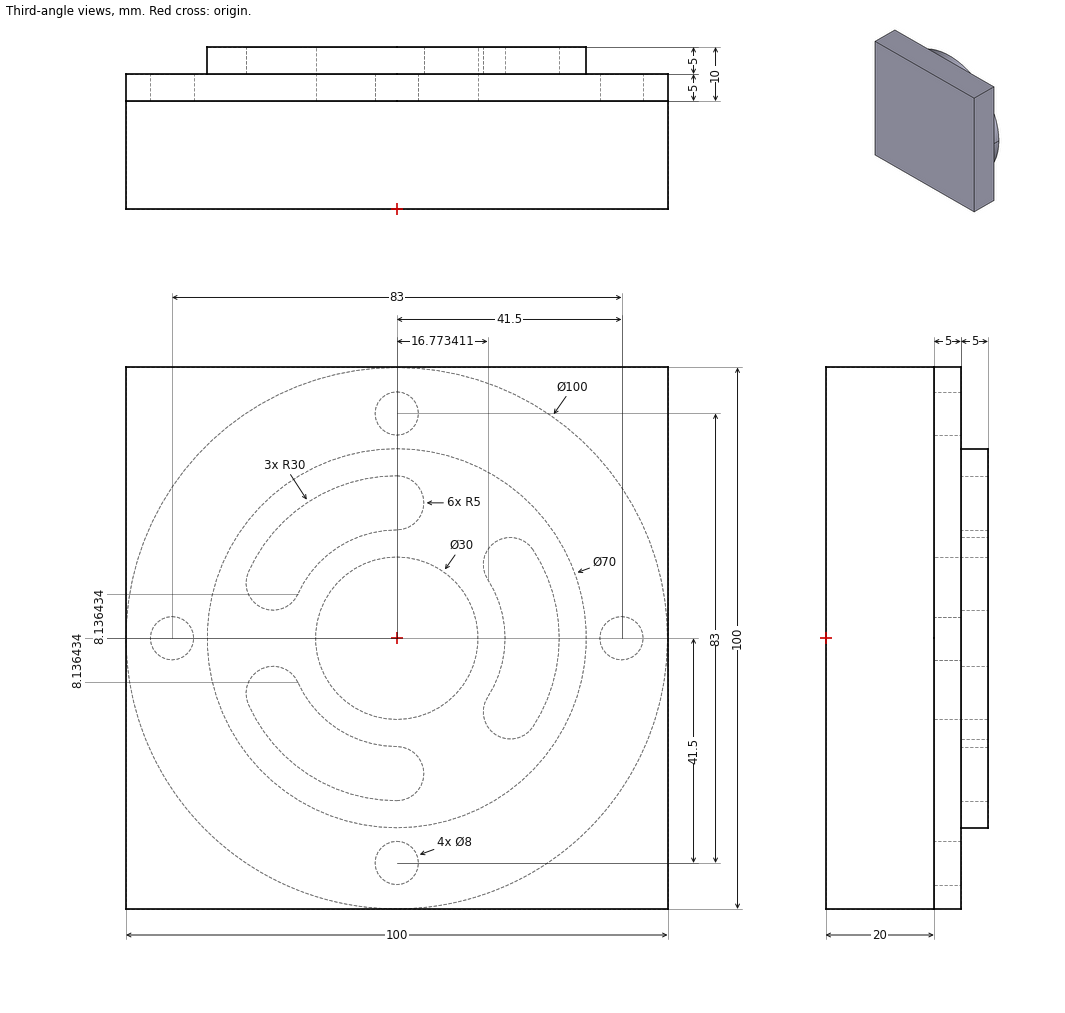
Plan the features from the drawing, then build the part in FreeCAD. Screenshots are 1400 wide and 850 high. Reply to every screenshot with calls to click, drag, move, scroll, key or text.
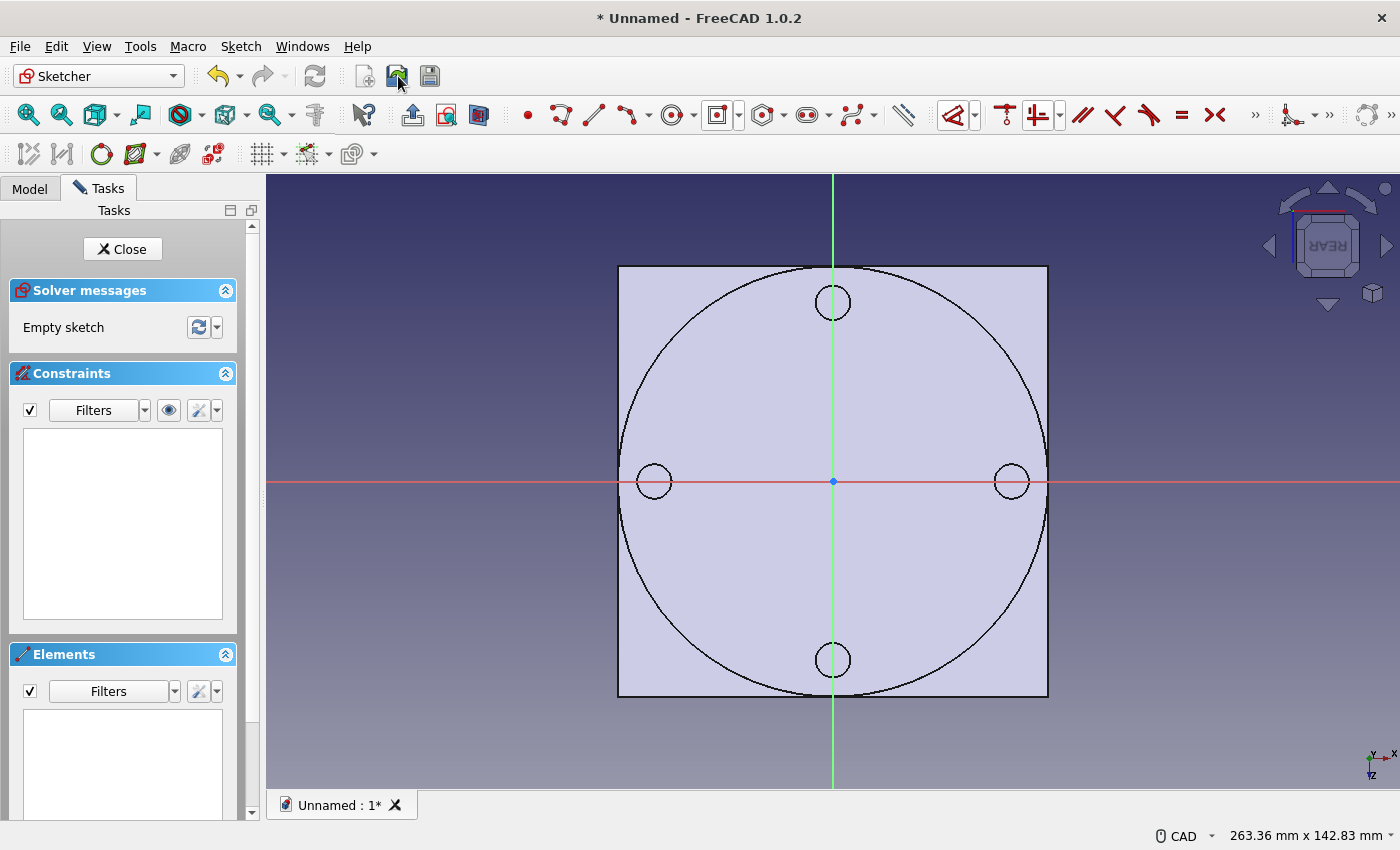
click(672, 116)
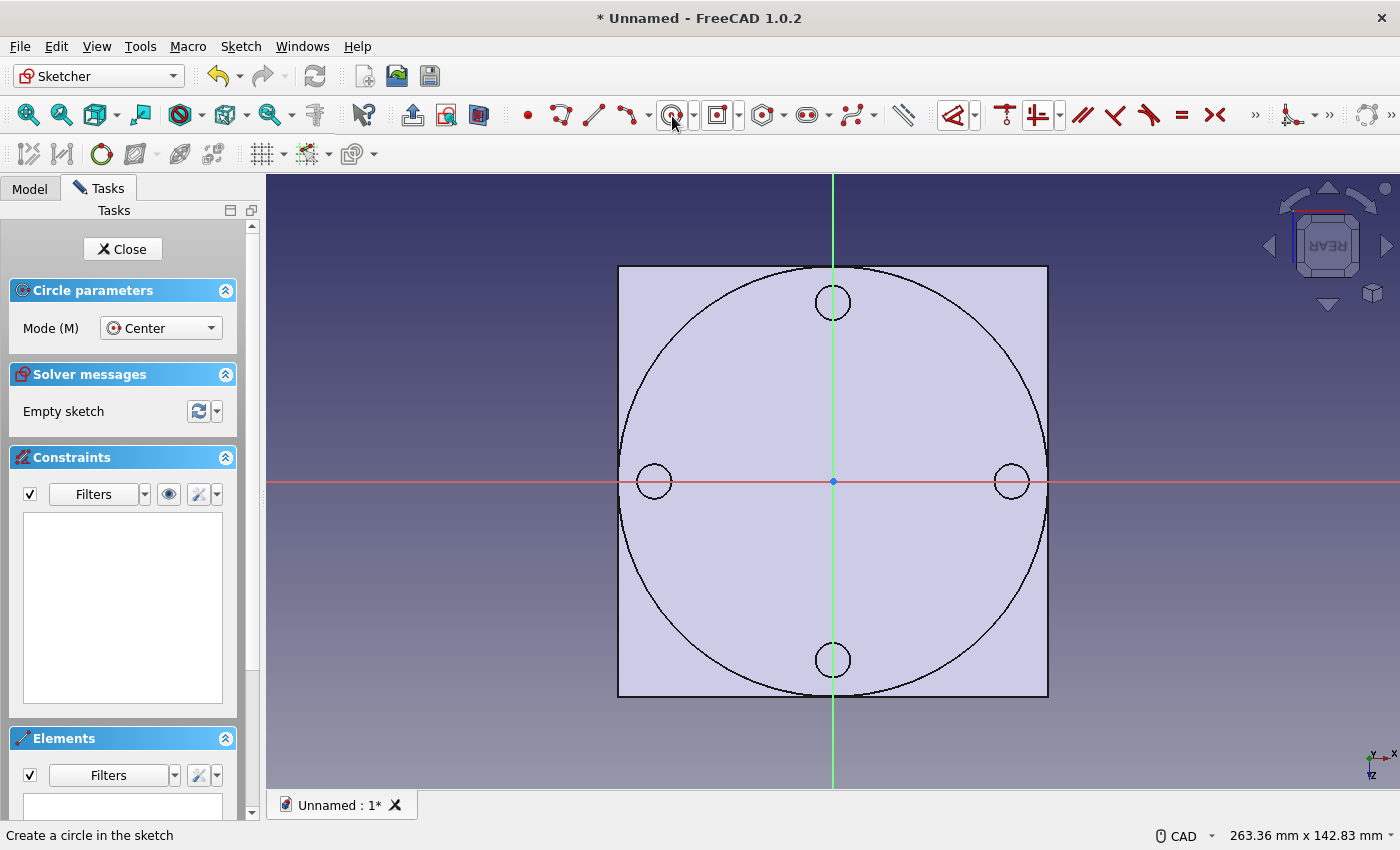
click(833, 481)
move(940, 375)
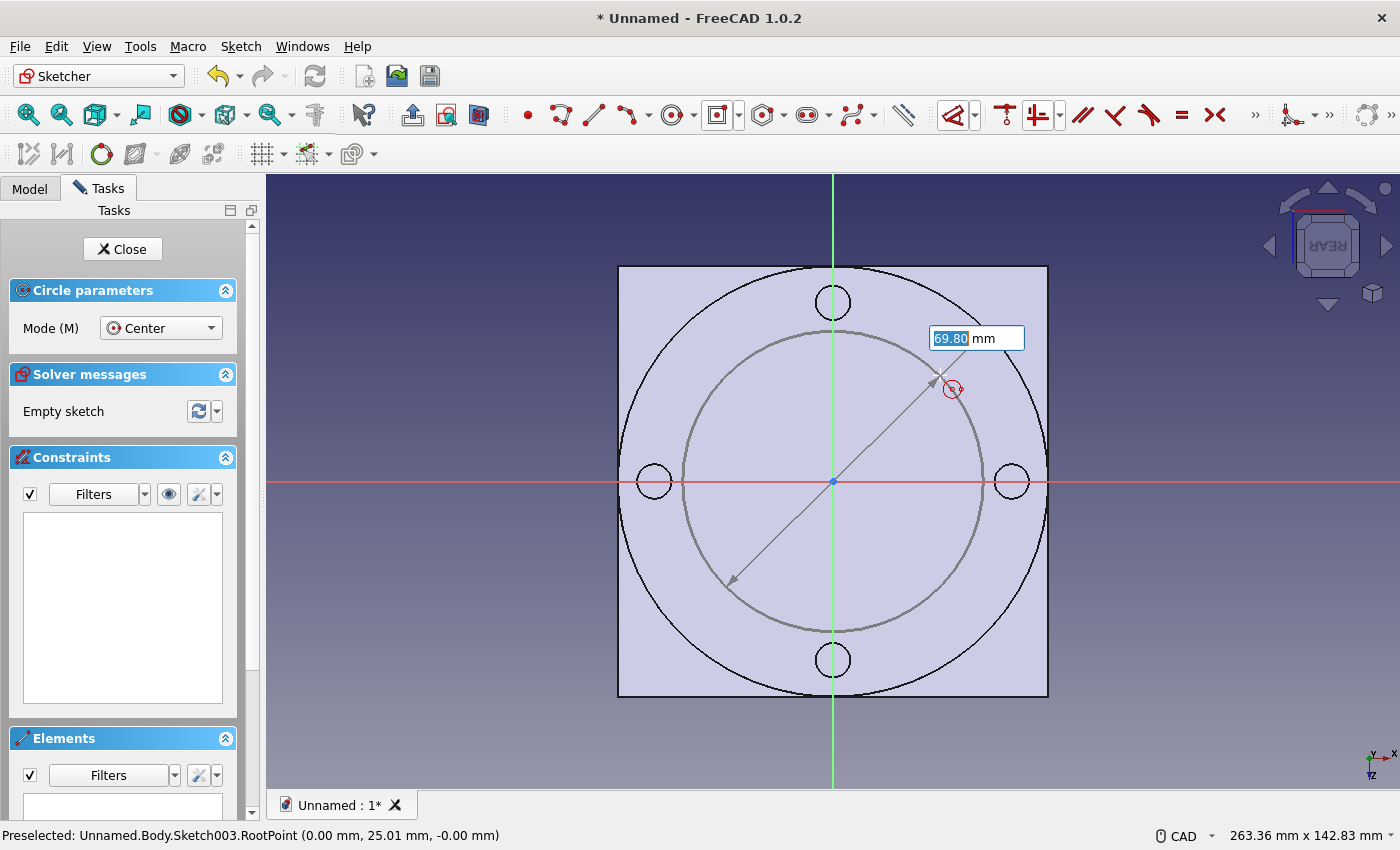
text(70)
key(Return)
key(Escape)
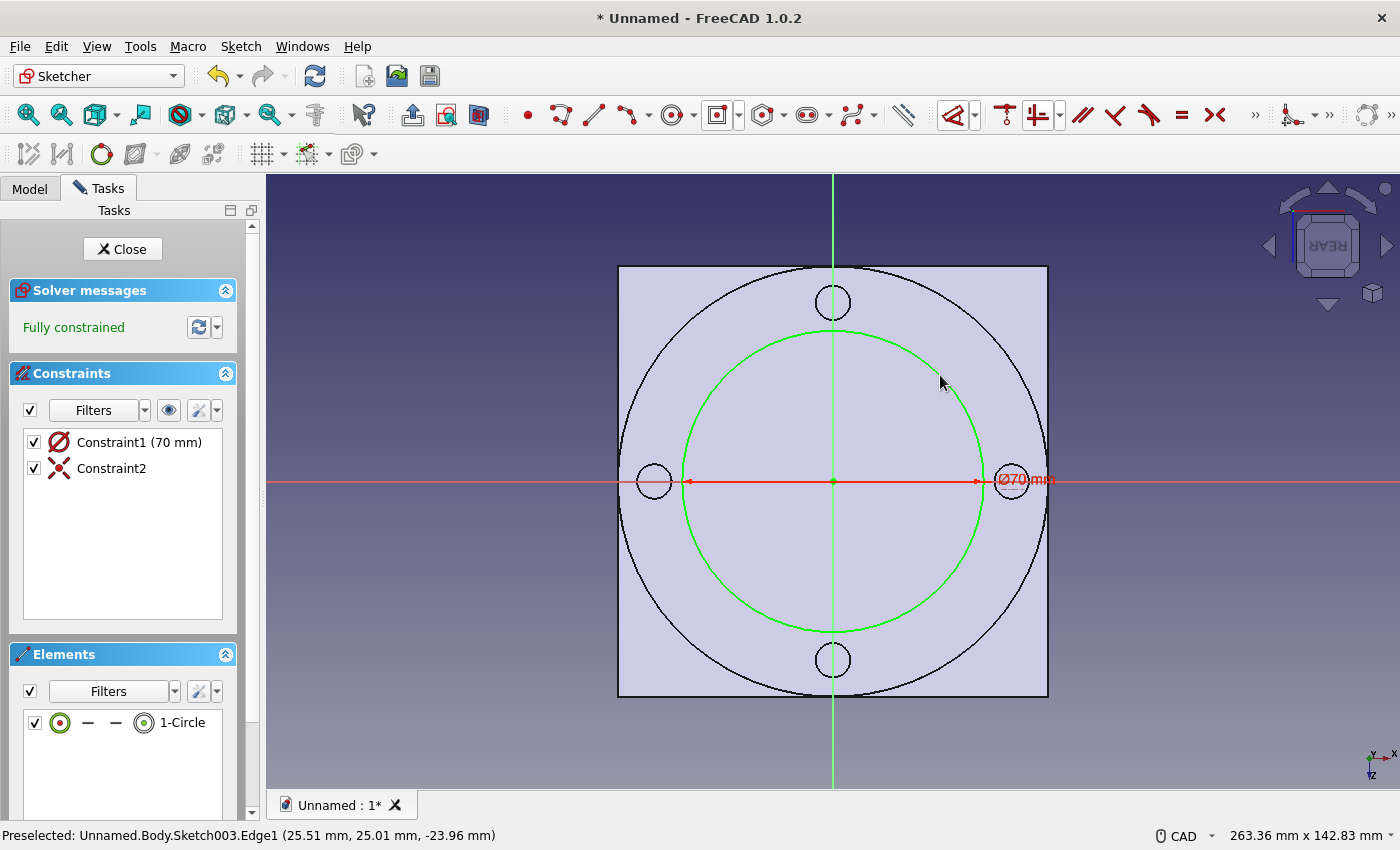
click(123, 249)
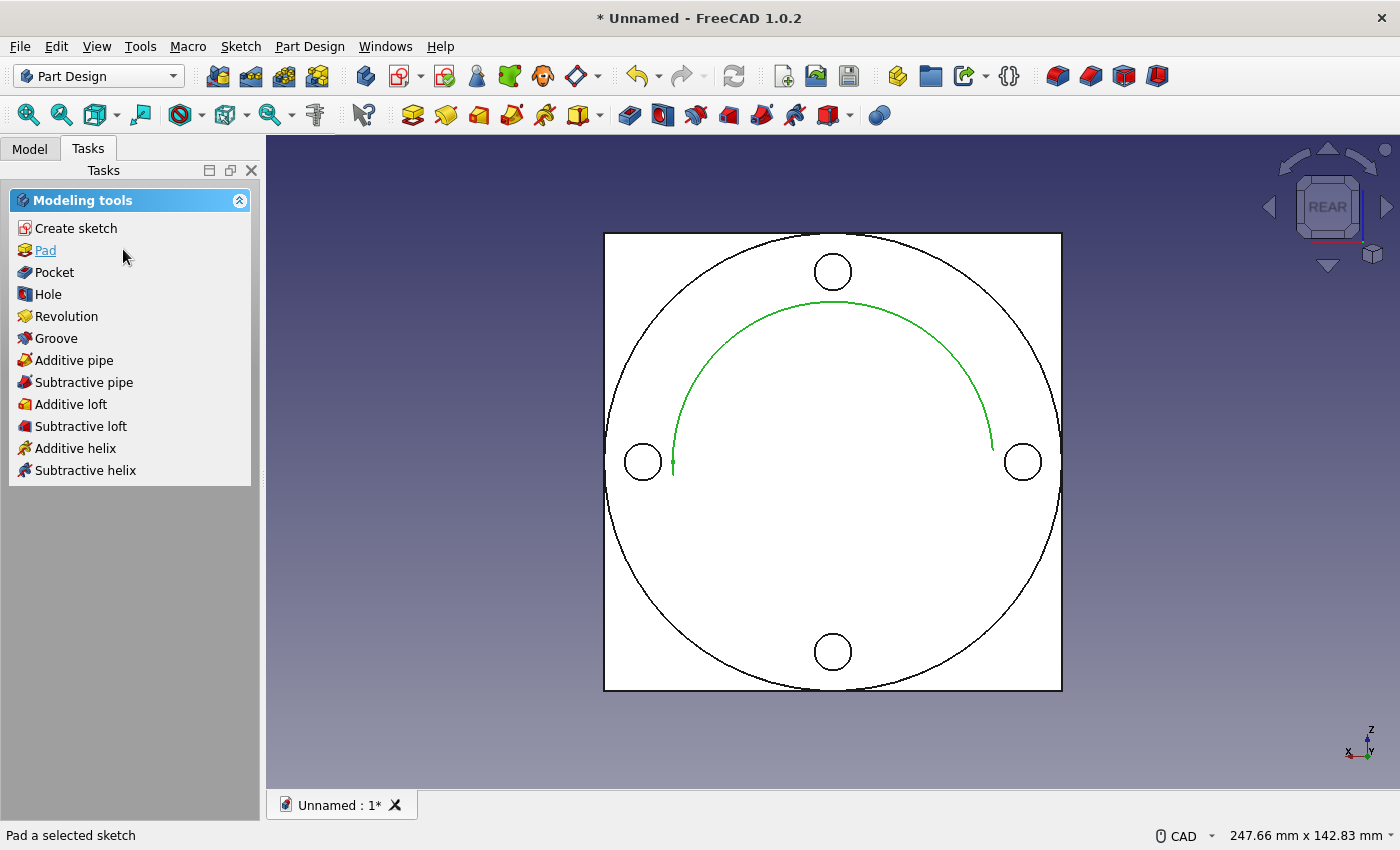
click(413, 116)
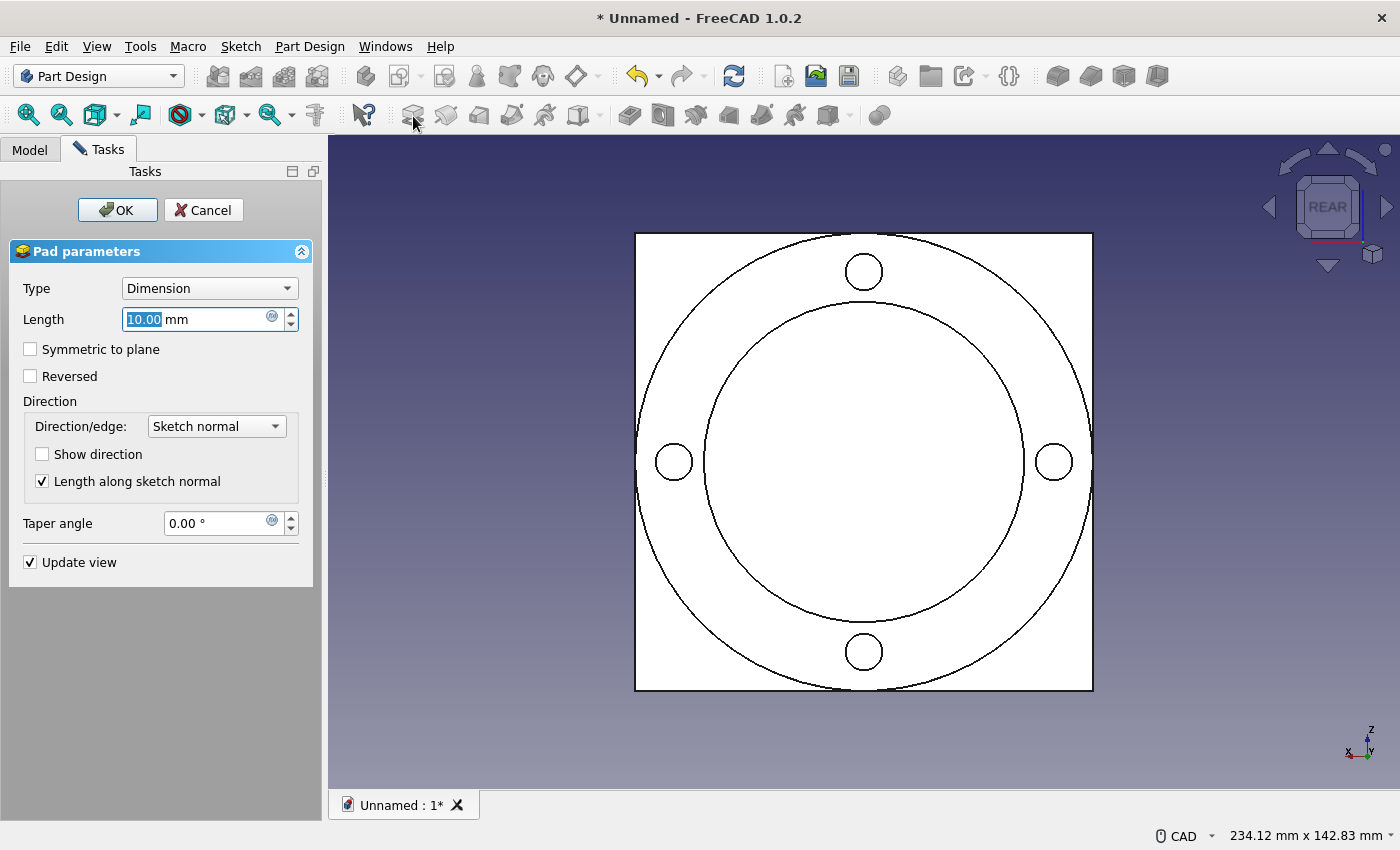
text(5)
key(Tab)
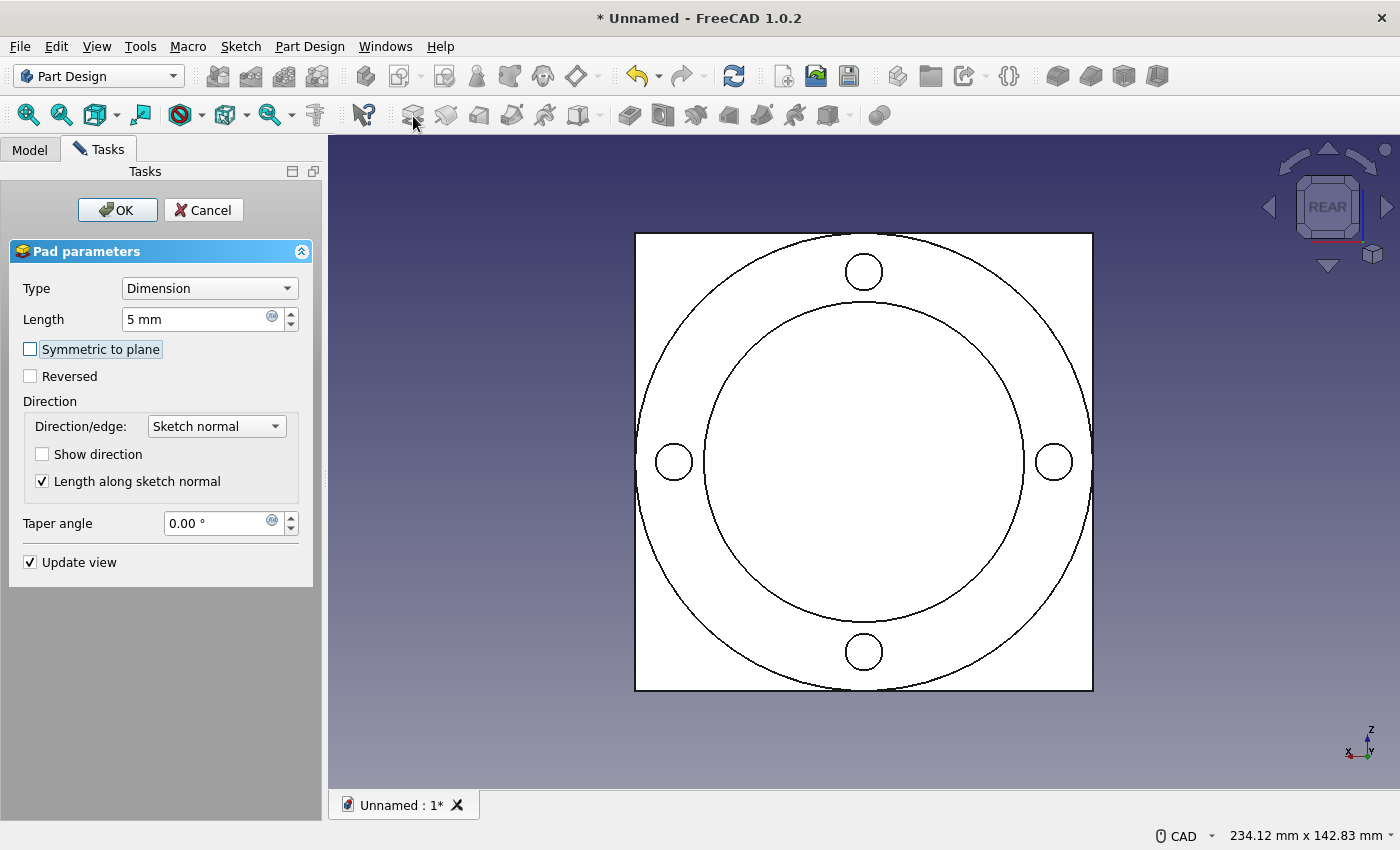
click(118, 210)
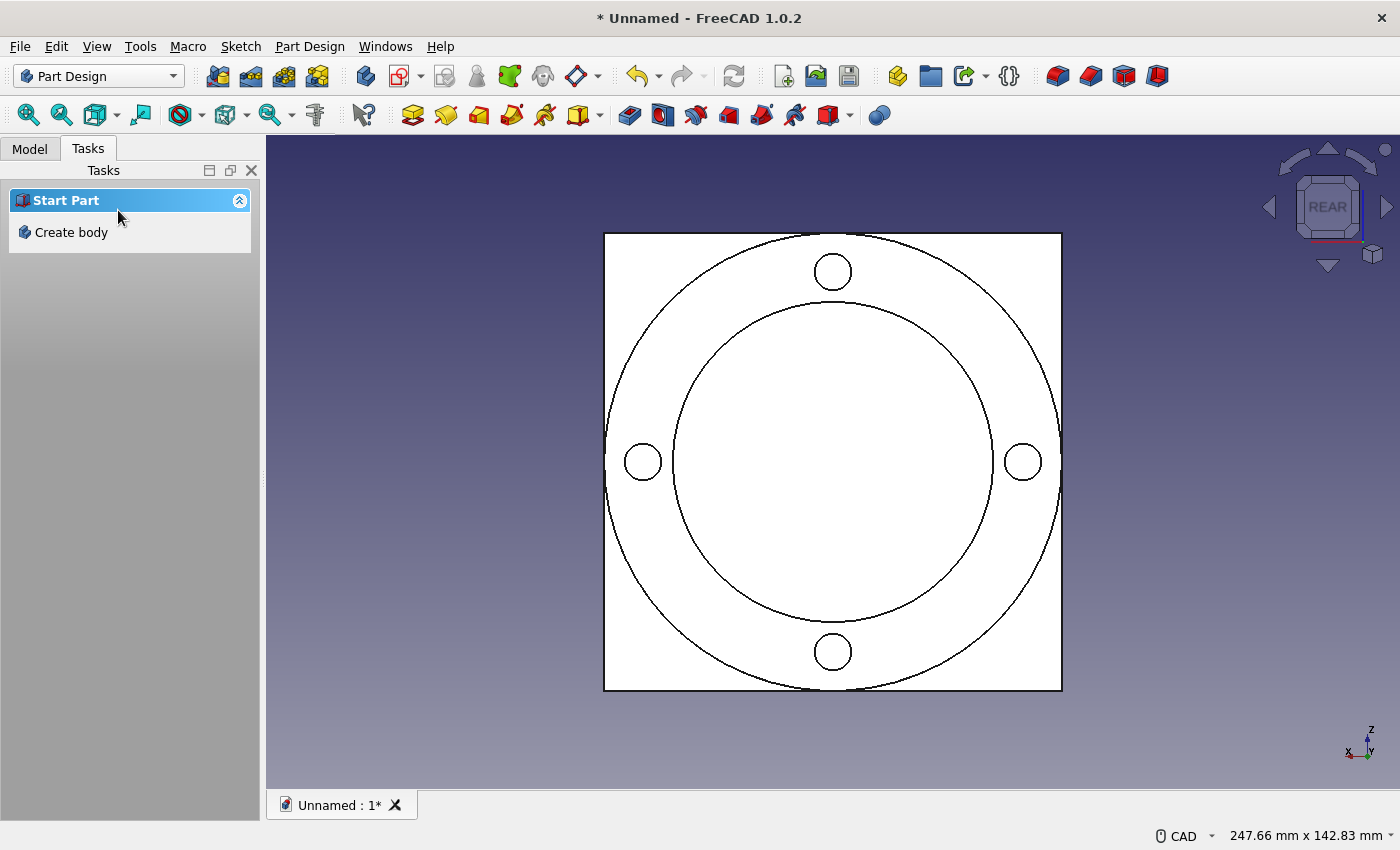
click(833, 461)